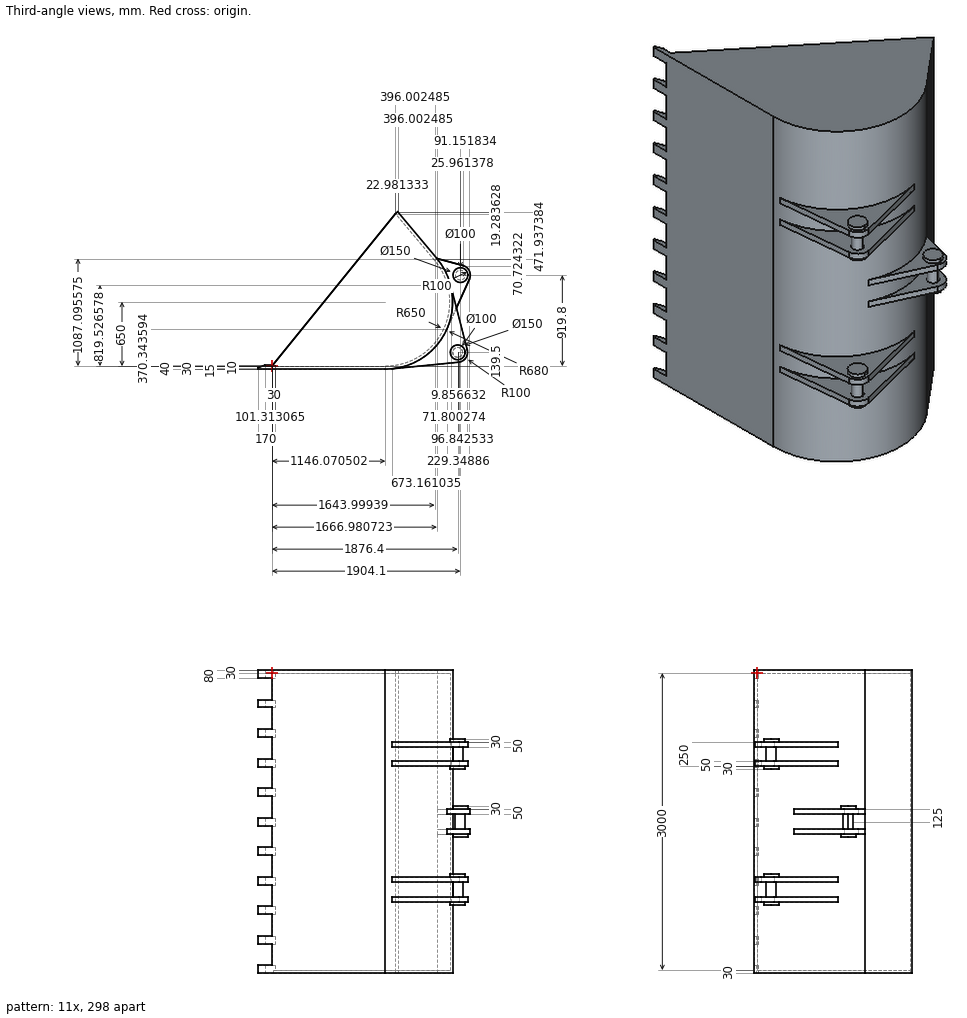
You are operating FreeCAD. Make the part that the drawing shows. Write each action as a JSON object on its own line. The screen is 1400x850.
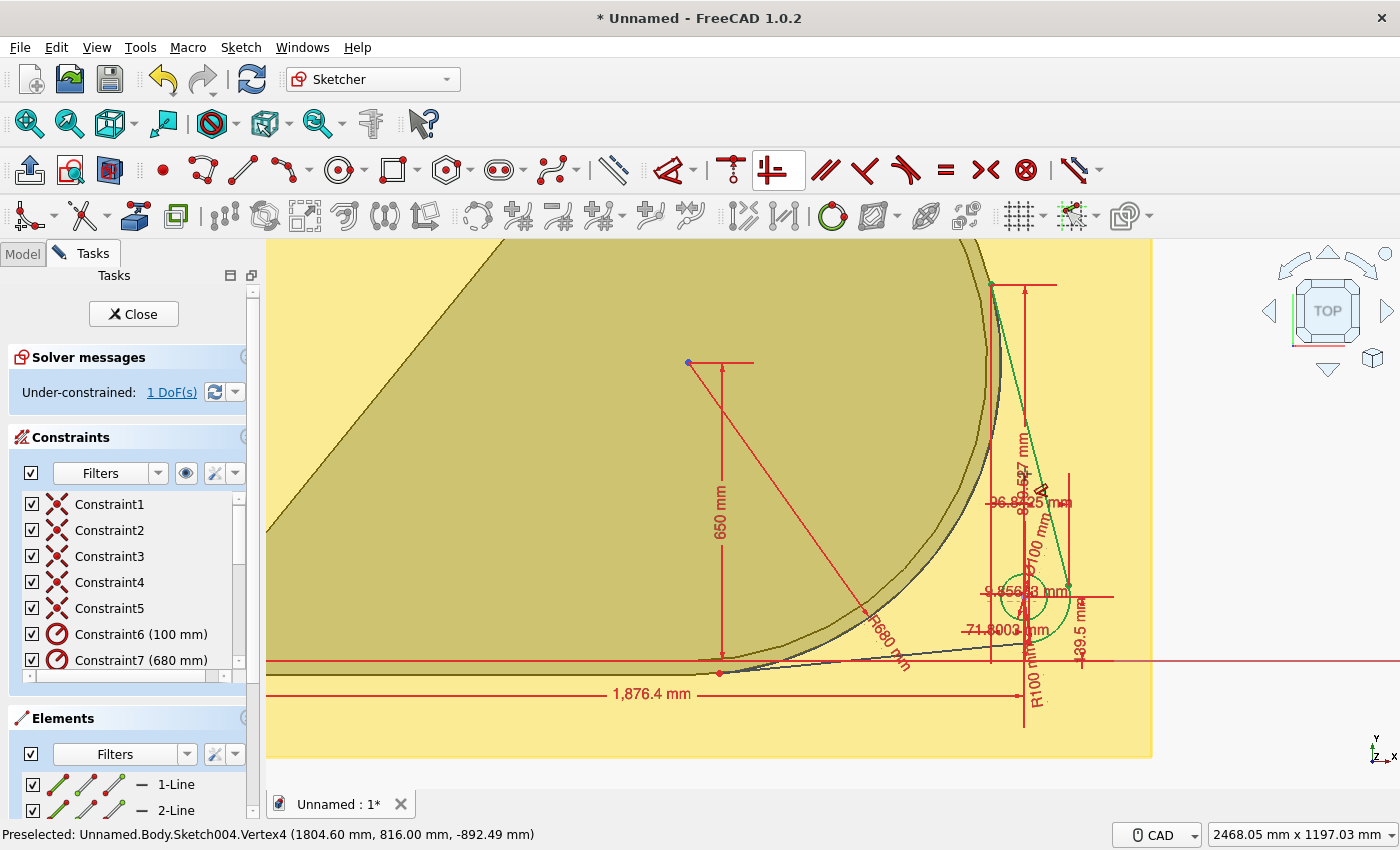
{"action": "left_click", "coordinate": [812, 664]}
{"action": "left_click", "coordinate": [874, 708]}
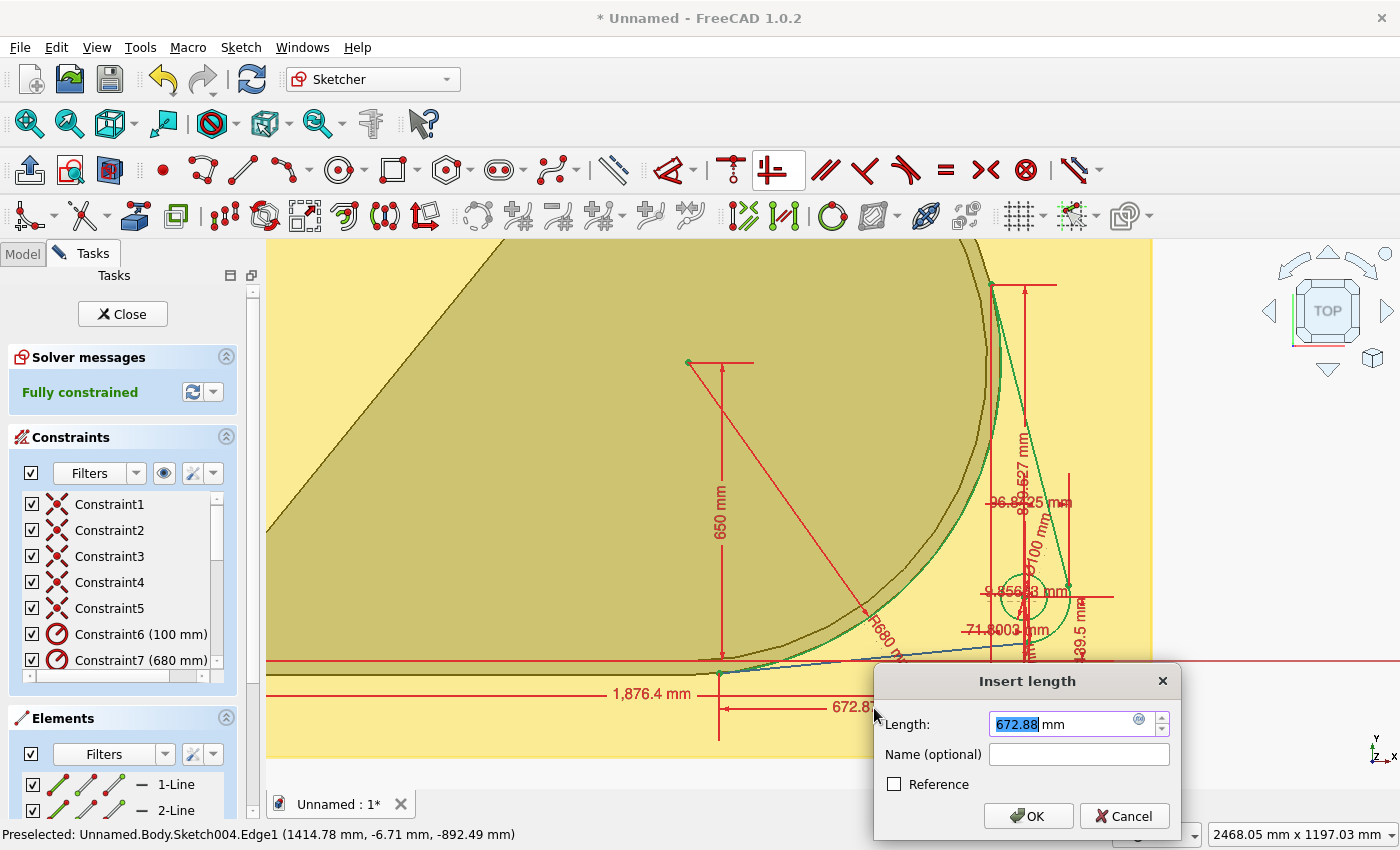
{"action": "type", "text": "673.161035"}
{"action": "key", "text": "Return"}
{"action": "key", "text": "Escape"}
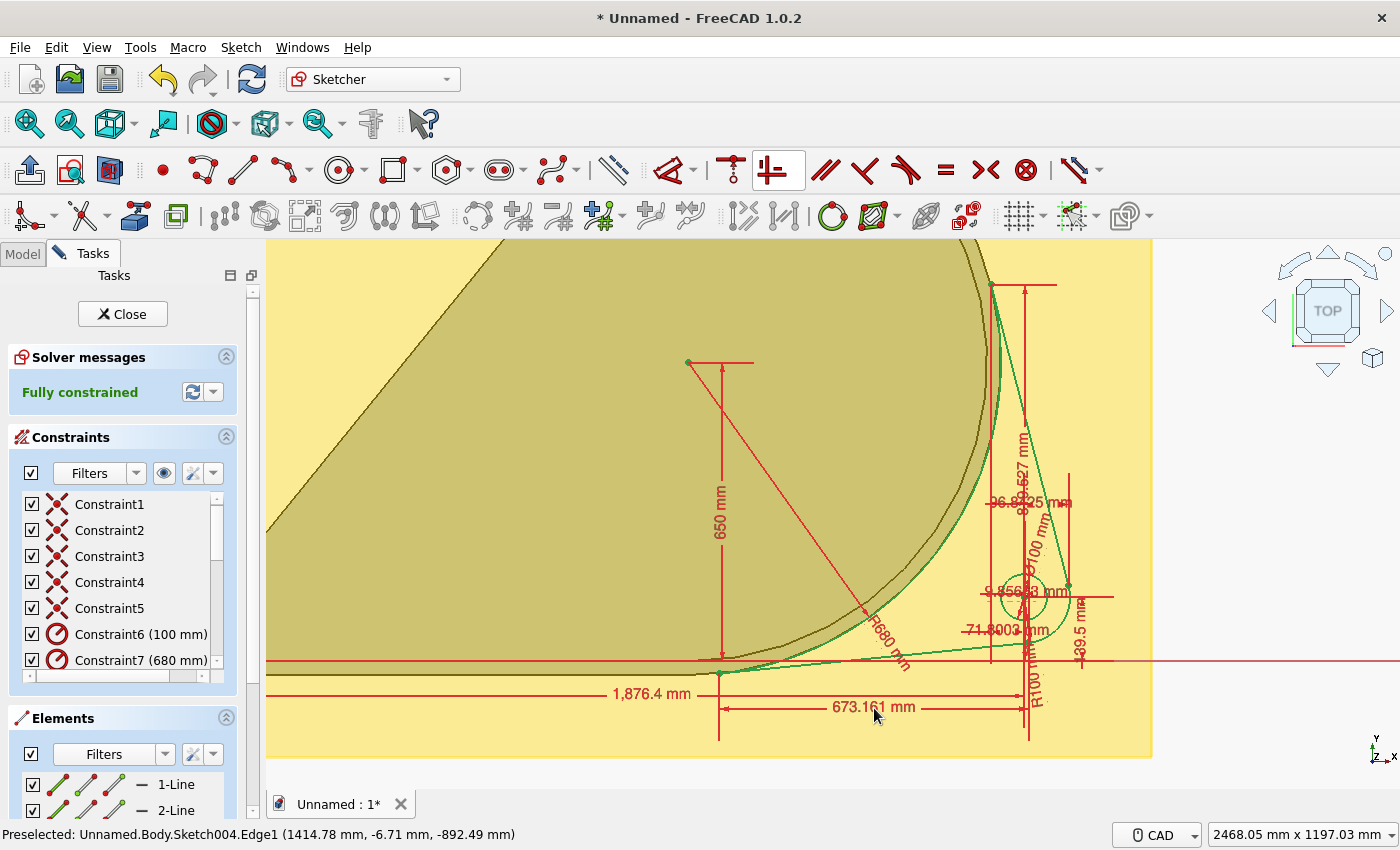
{"action": "left_click", "coordinate": [123, 314]}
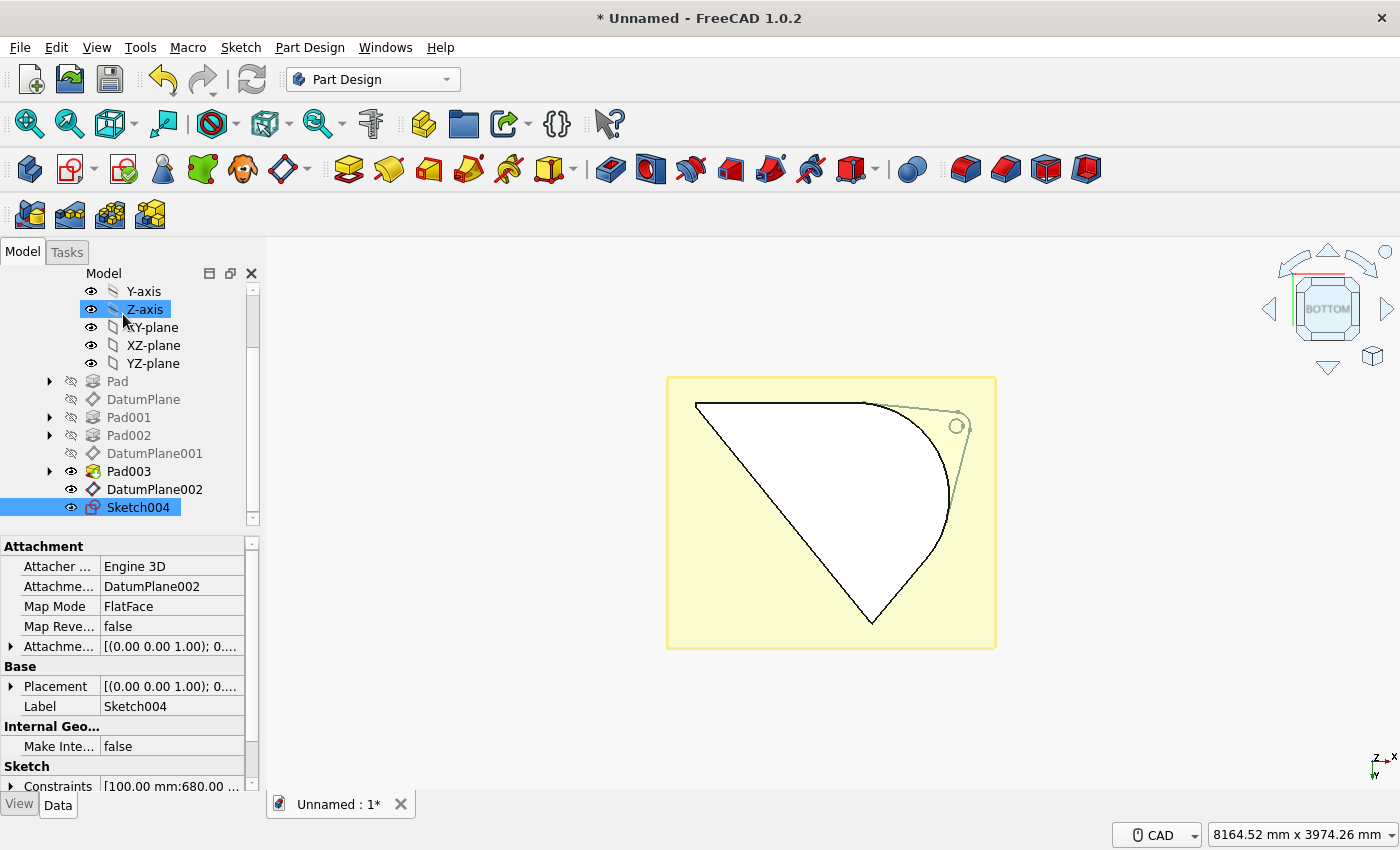
{"action": "left_click", "coordinate": [350, 170]}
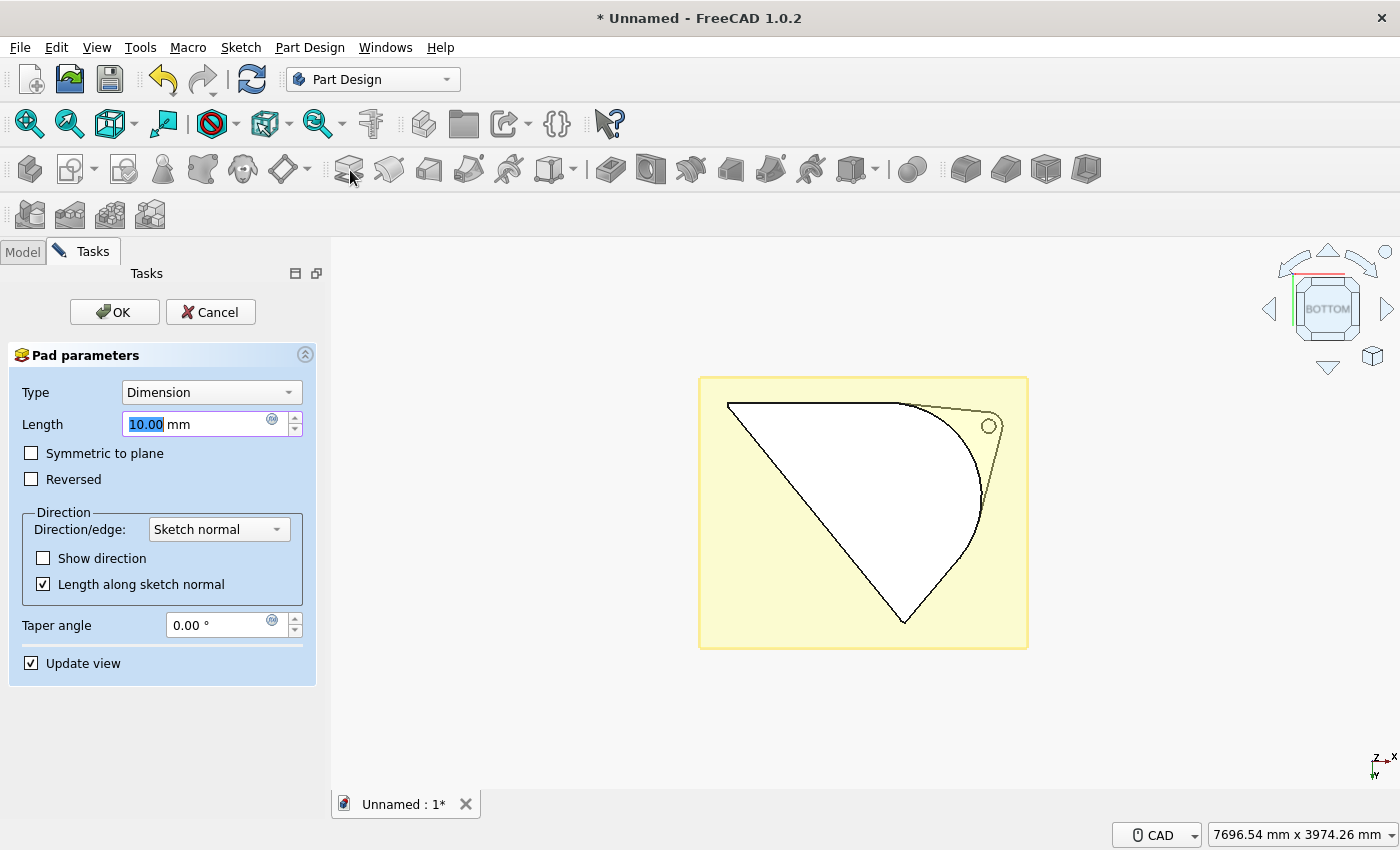
{"action": "type", "text": "50"}
{"action": "key", "text": "Tab"}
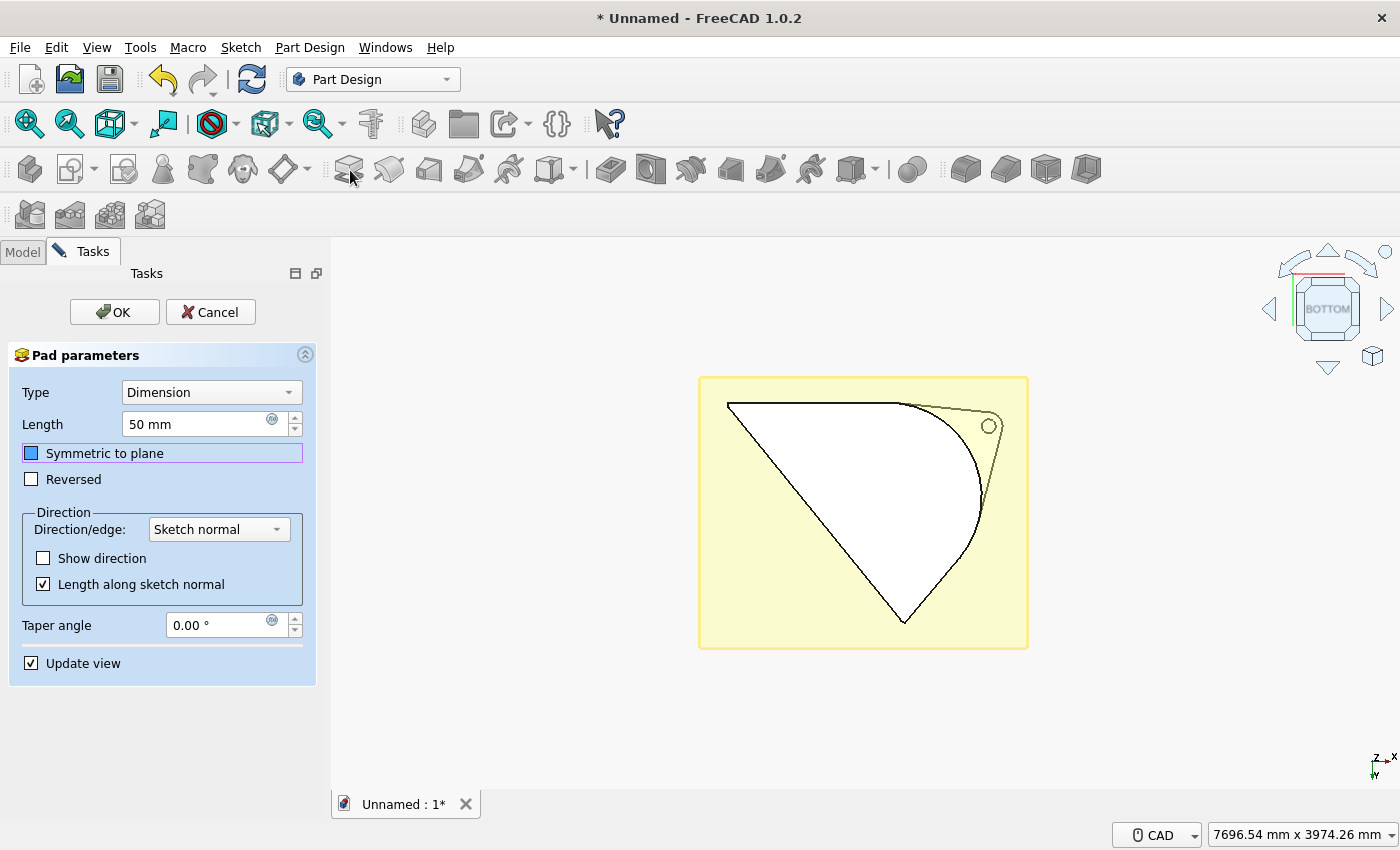
{"action": "left_click", "coordinate": [30, 479]}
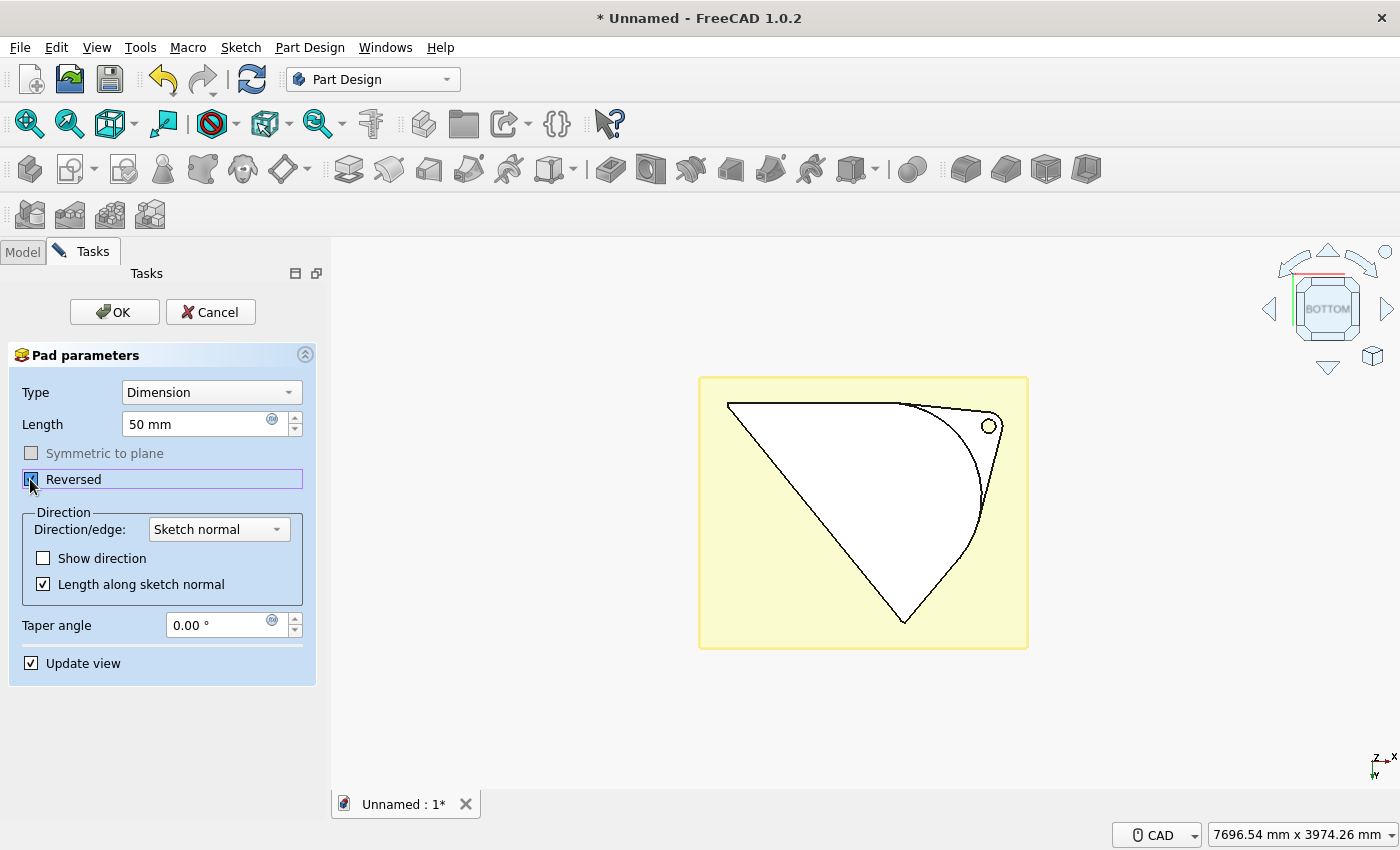
{"action": "left_click", "coordinate": [115, 312]}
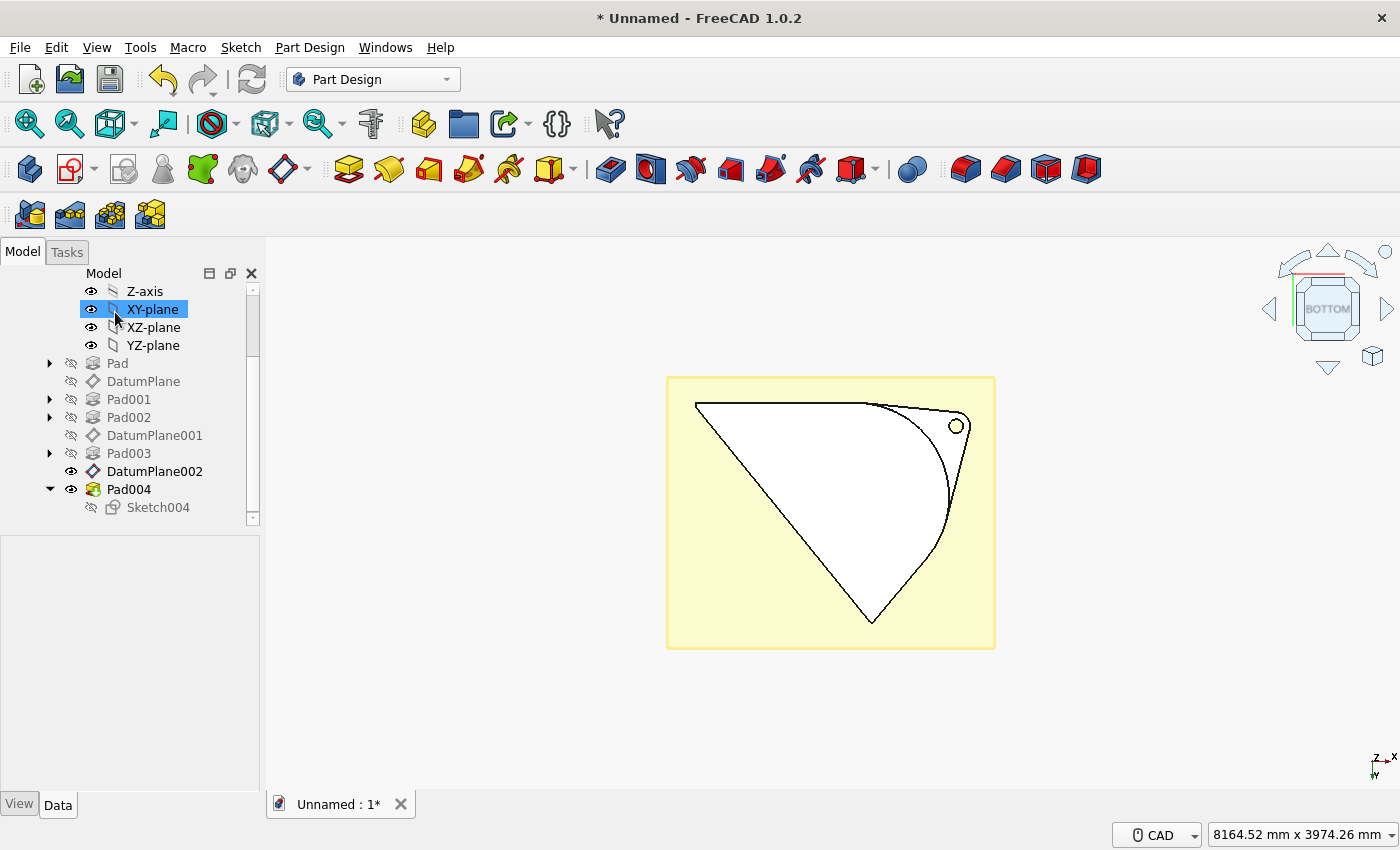
{"action": "left_click", "coordinate": [116, 471]}
{"action": "key", "text": "space"}